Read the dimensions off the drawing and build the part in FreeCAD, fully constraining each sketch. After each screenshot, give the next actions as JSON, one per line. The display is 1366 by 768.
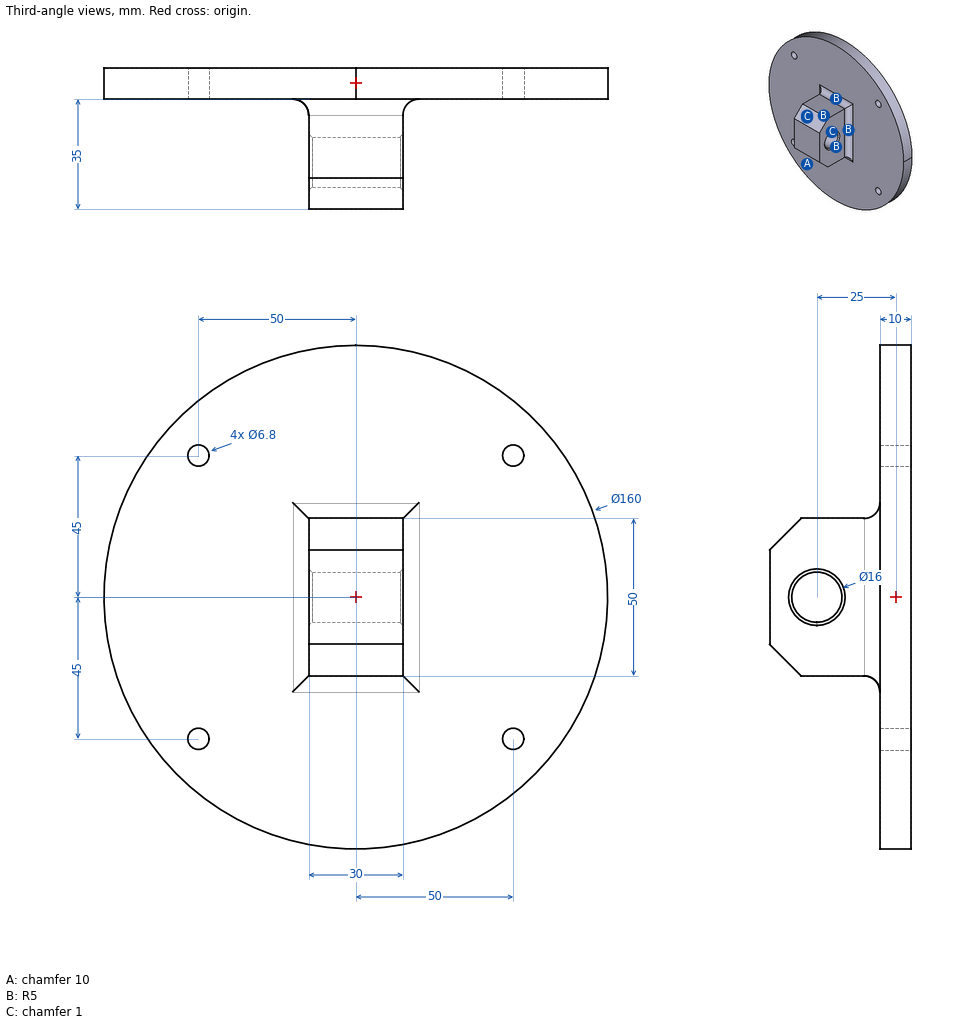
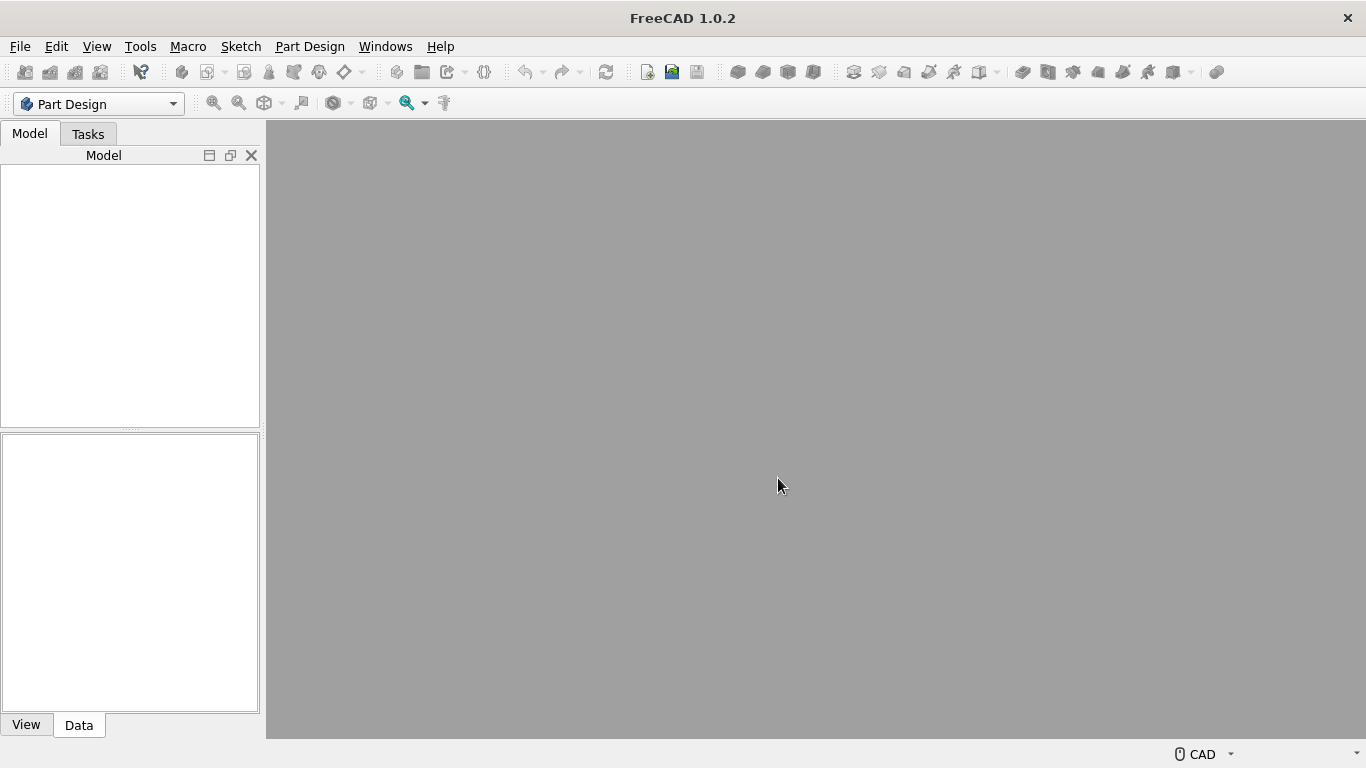
{"action": "key", "text": "ctrl+n"}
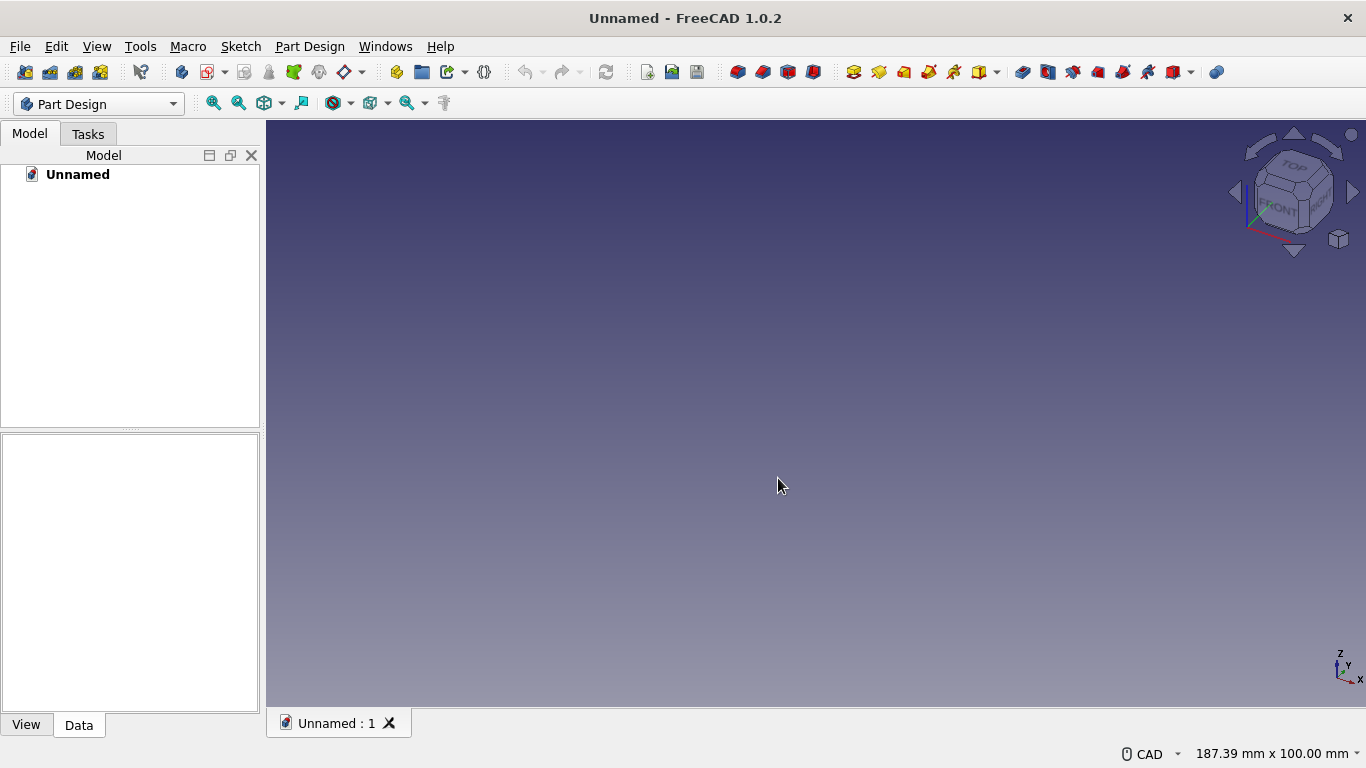
{"action": "left_click", "coordinate": [206, 72]}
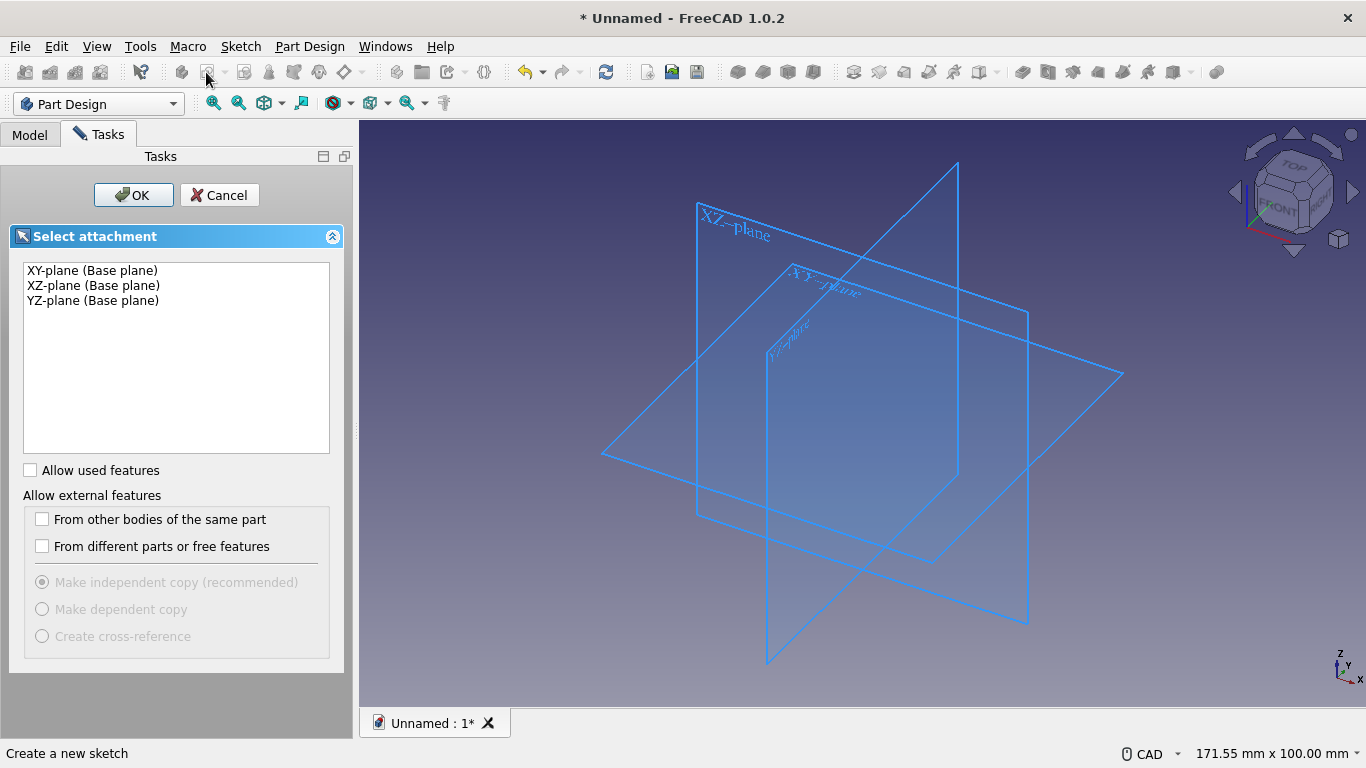
{"action": "left_click", "coordinate": [84, 286]}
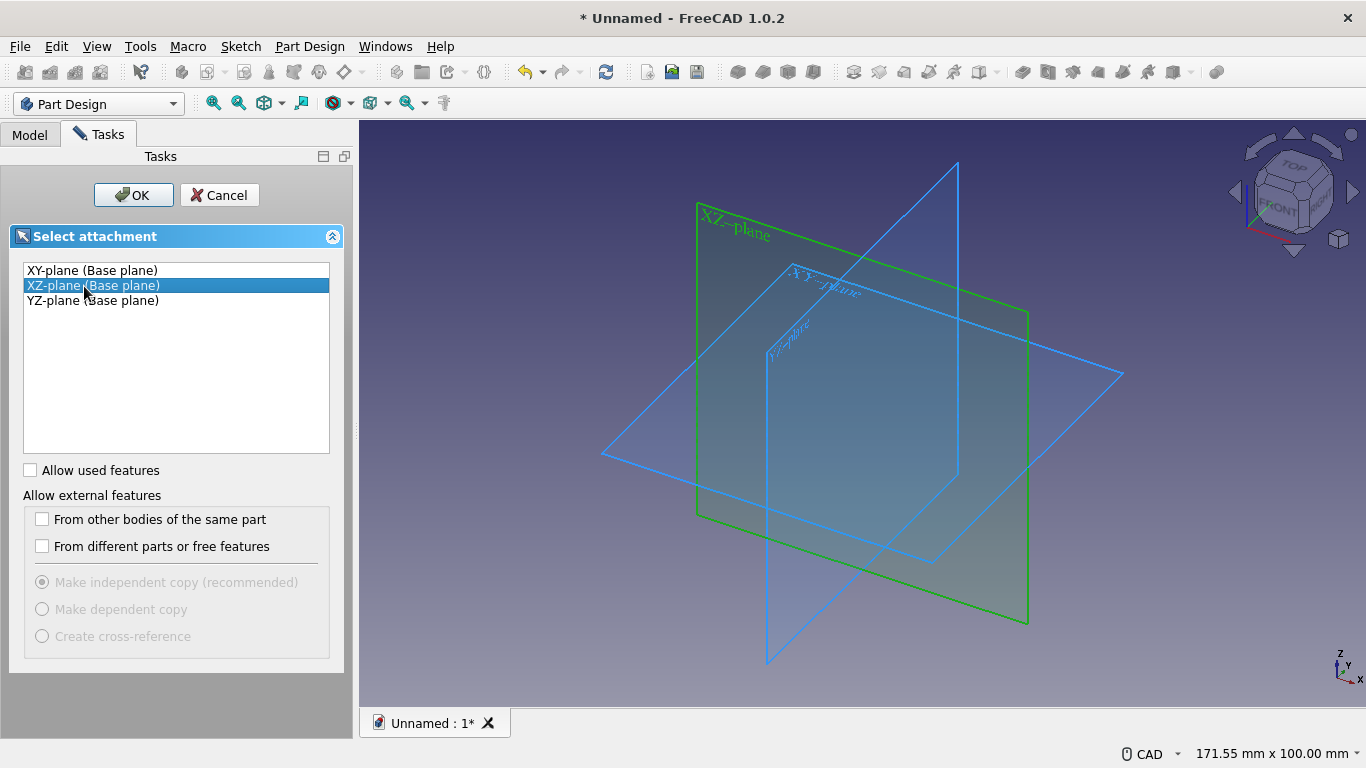
{"action": "left_click", "coordinate": [134, 195]}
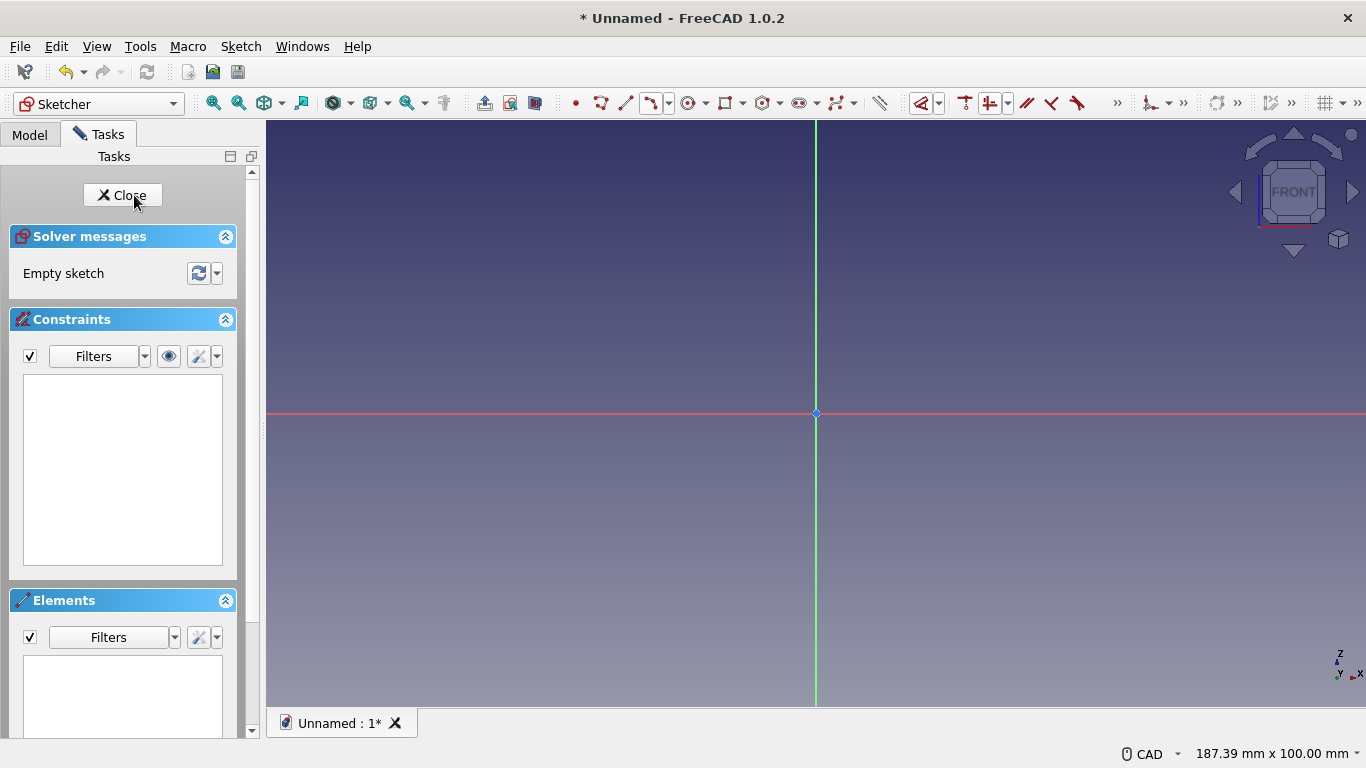
{"action": "scroll", "coordinate": [708, 414], "scroll_direction": "down", "scroll_amount": 5}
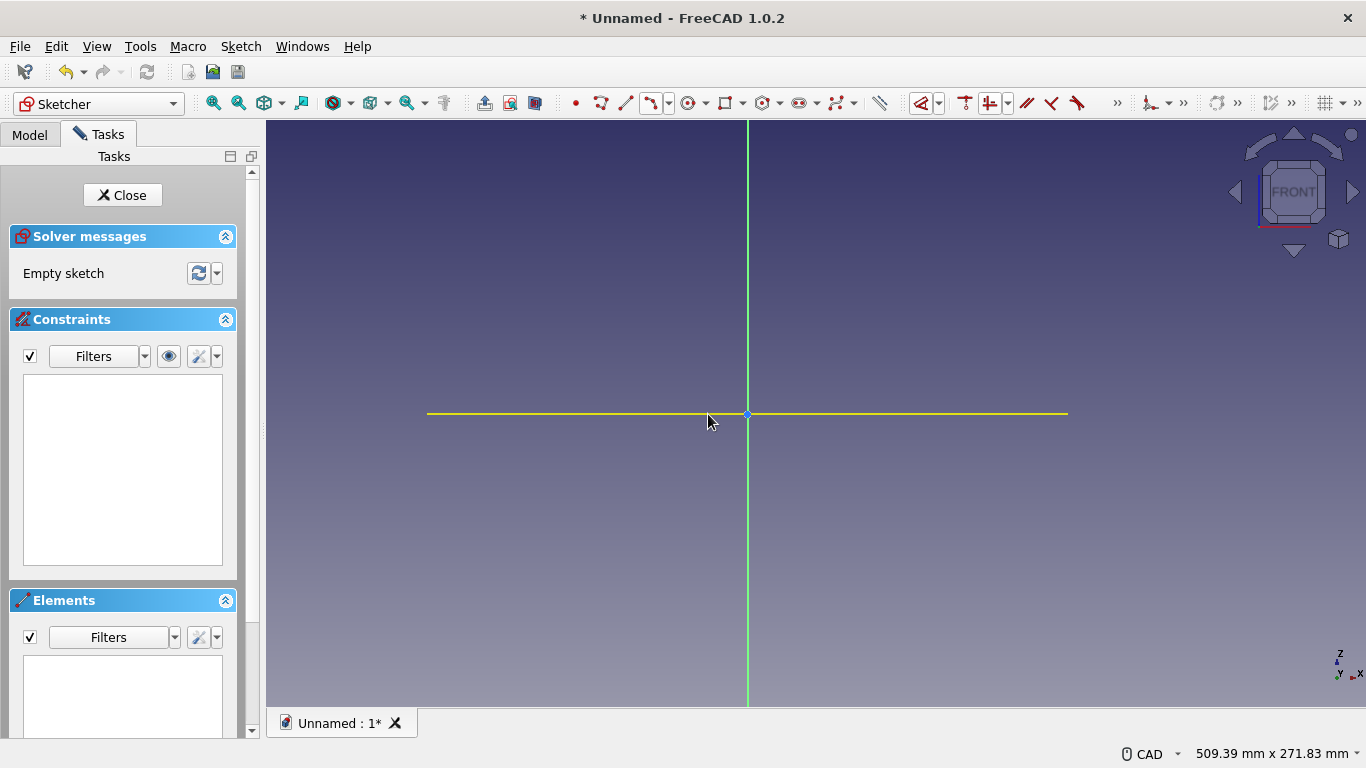
{"action": "key", "text": "g c"}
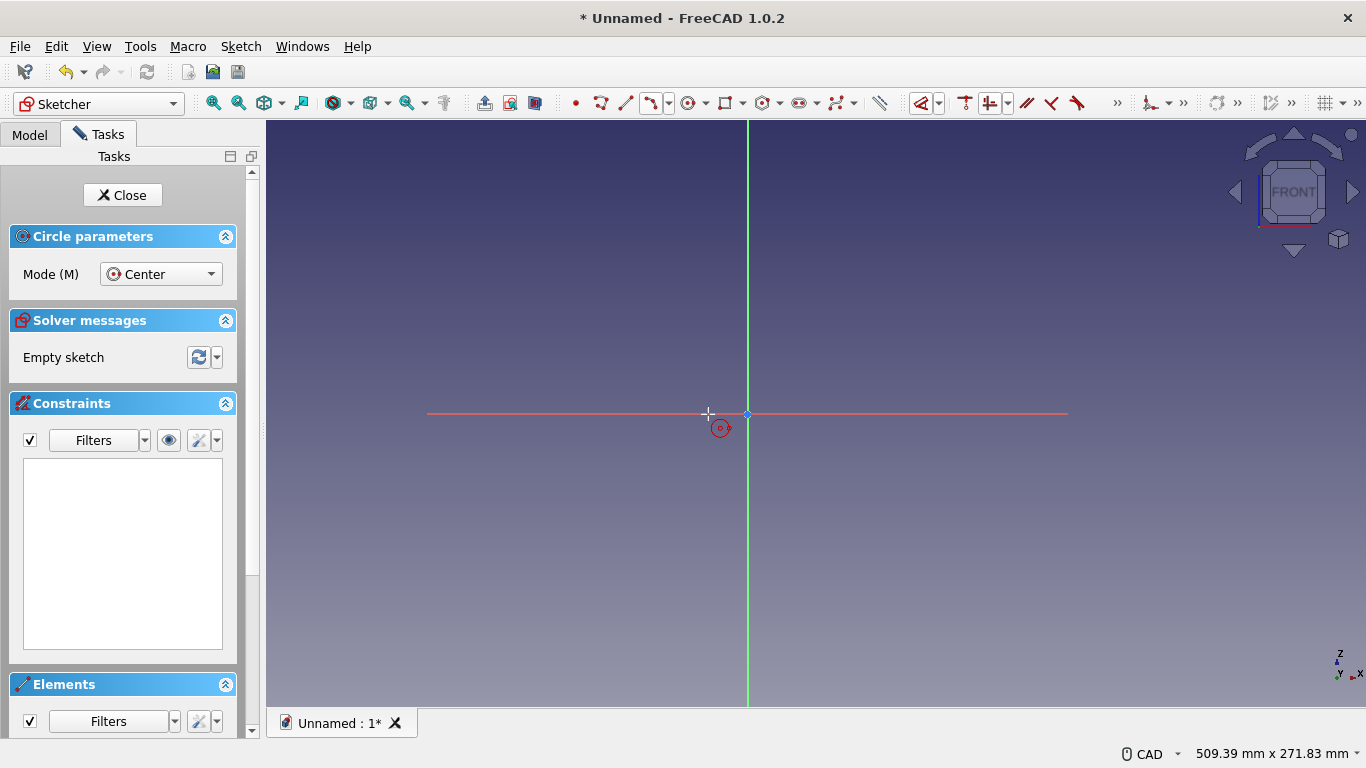
{"action": "left_click", "coordinate": [748, 414]}
{"action": "left_click", "coordinate": [870, 292]}
{"action": "key", "text": "Escape"}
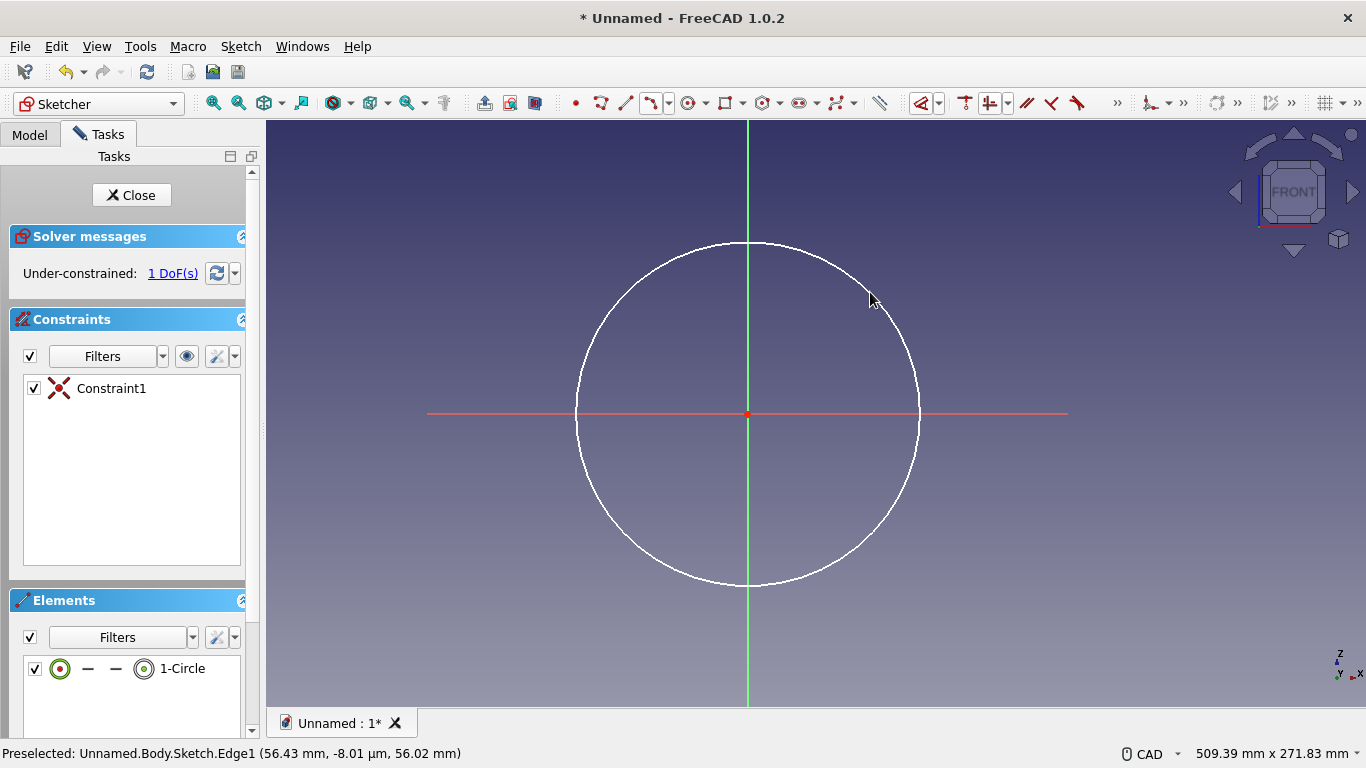
{"action": "key", "text": "d"}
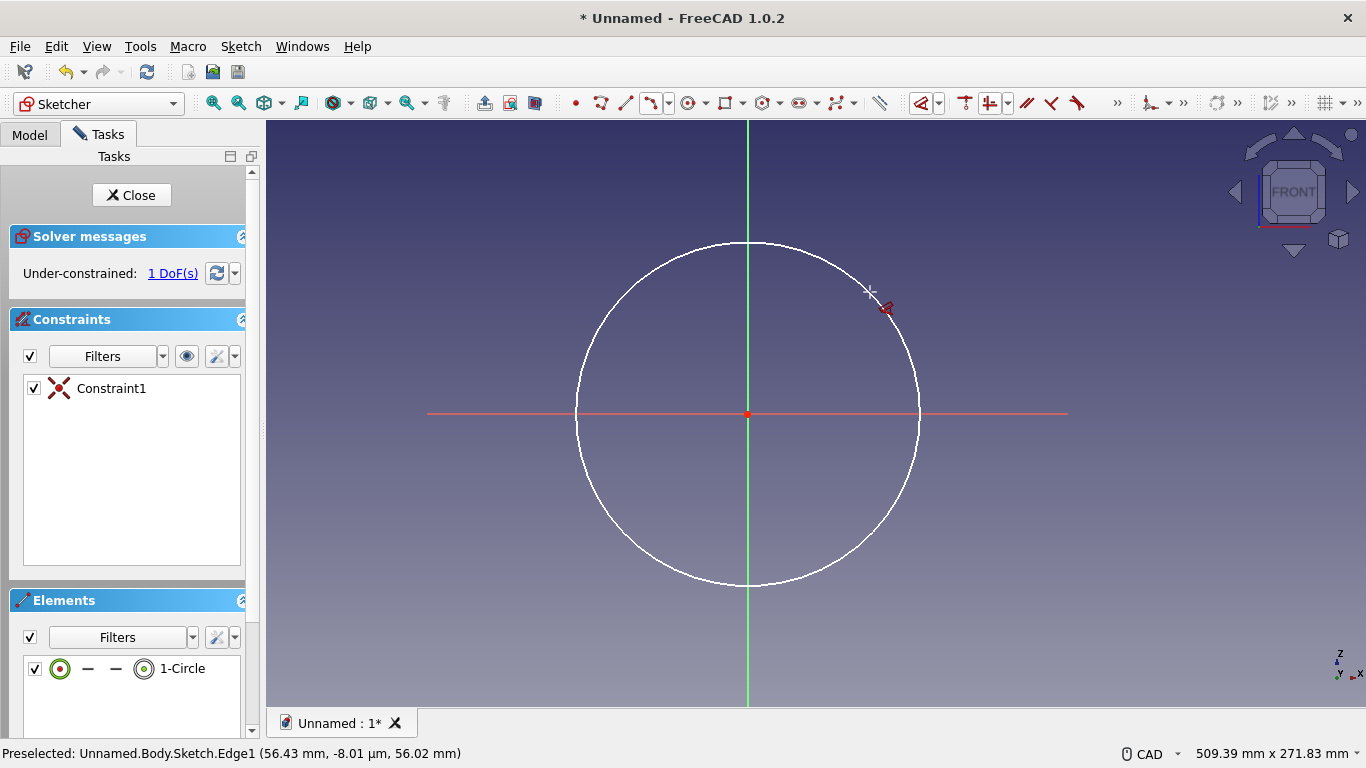
{"action": "left_click", "coordinate": [869, 292]}
{"action": "left_click", "coordinate": [892, 269]}